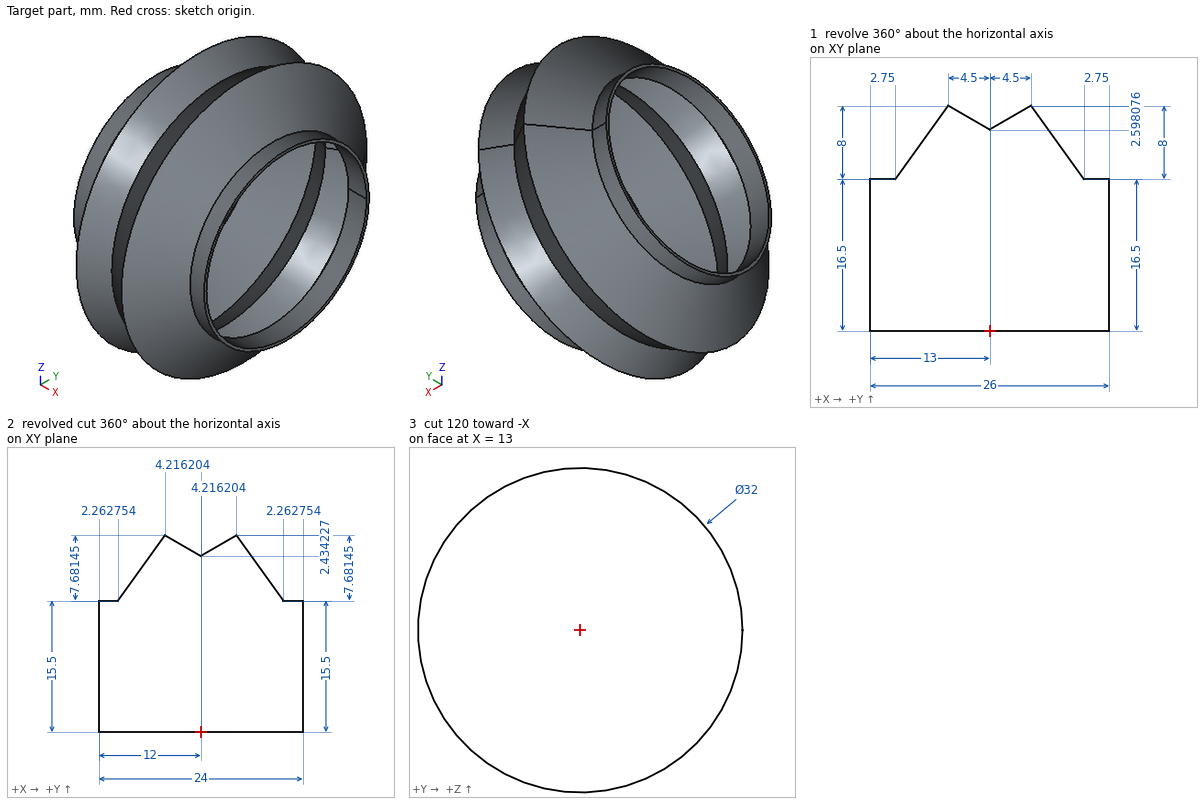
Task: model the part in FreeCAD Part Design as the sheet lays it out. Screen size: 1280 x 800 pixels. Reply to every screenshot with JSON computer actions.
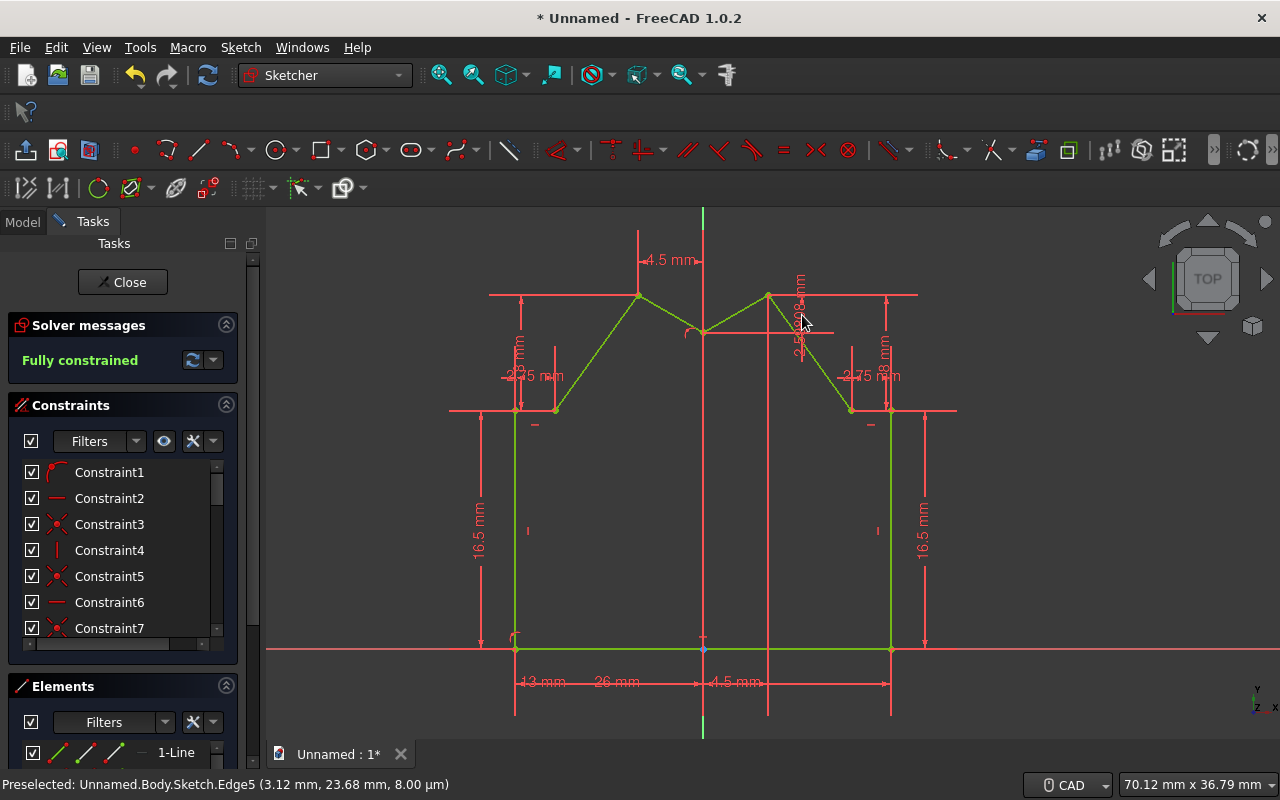
{"action": "left_click", "coordinate": [123, 282]}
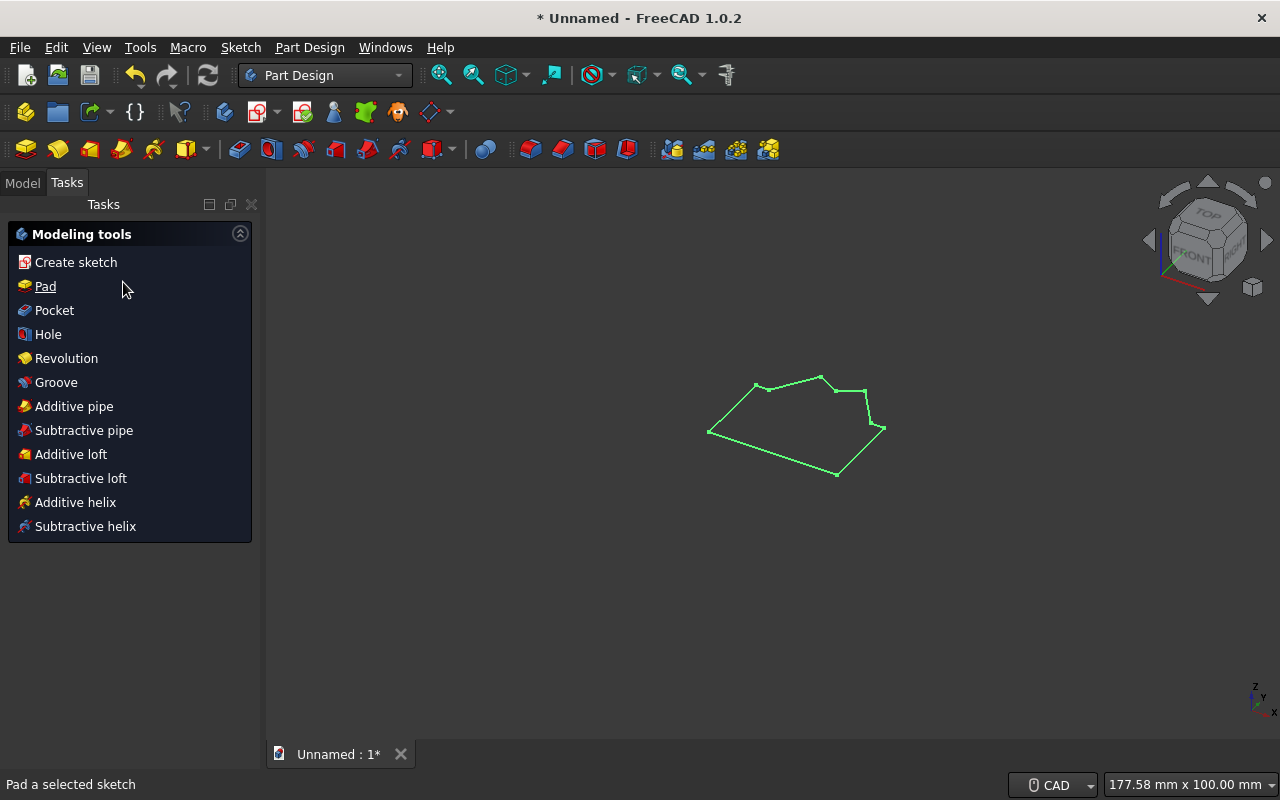
{"action": "left_click", "coordinate": [58, 150]}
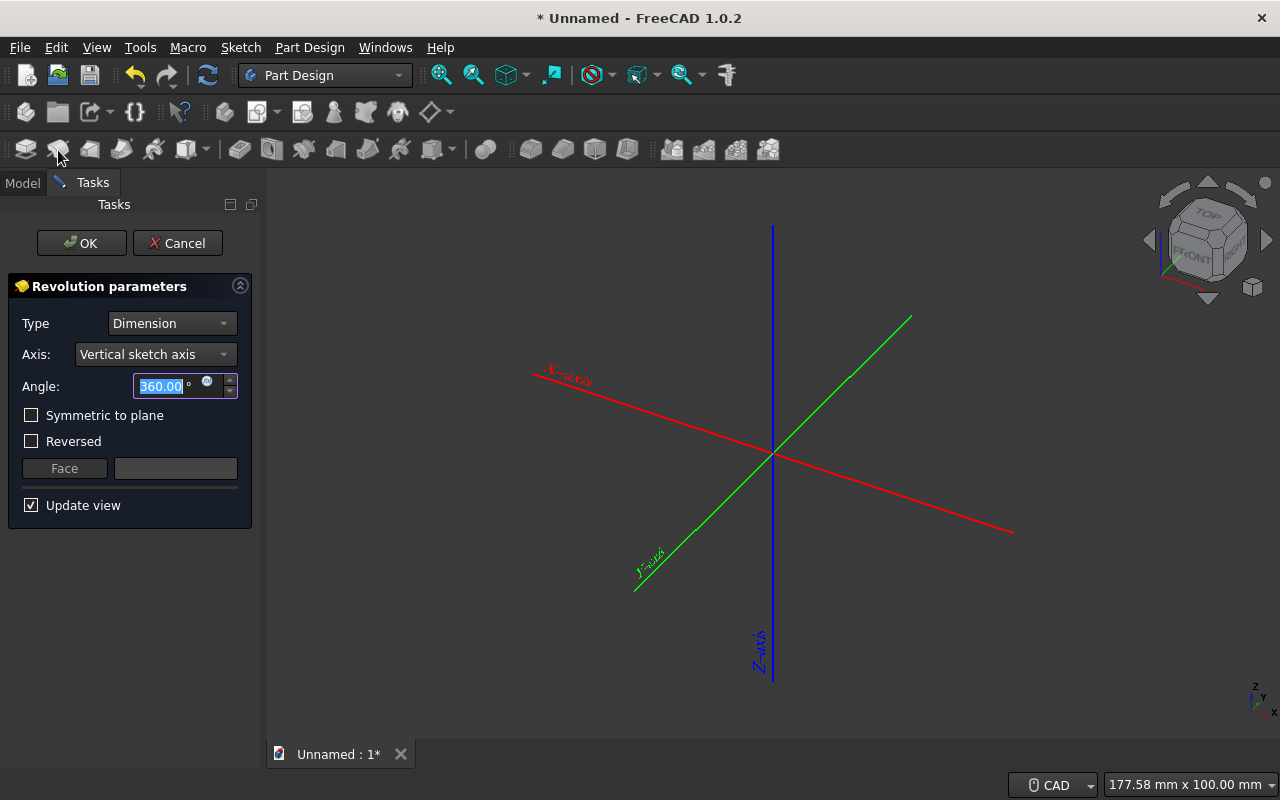
{"action": "left_click", "coordinate": [156, 354]}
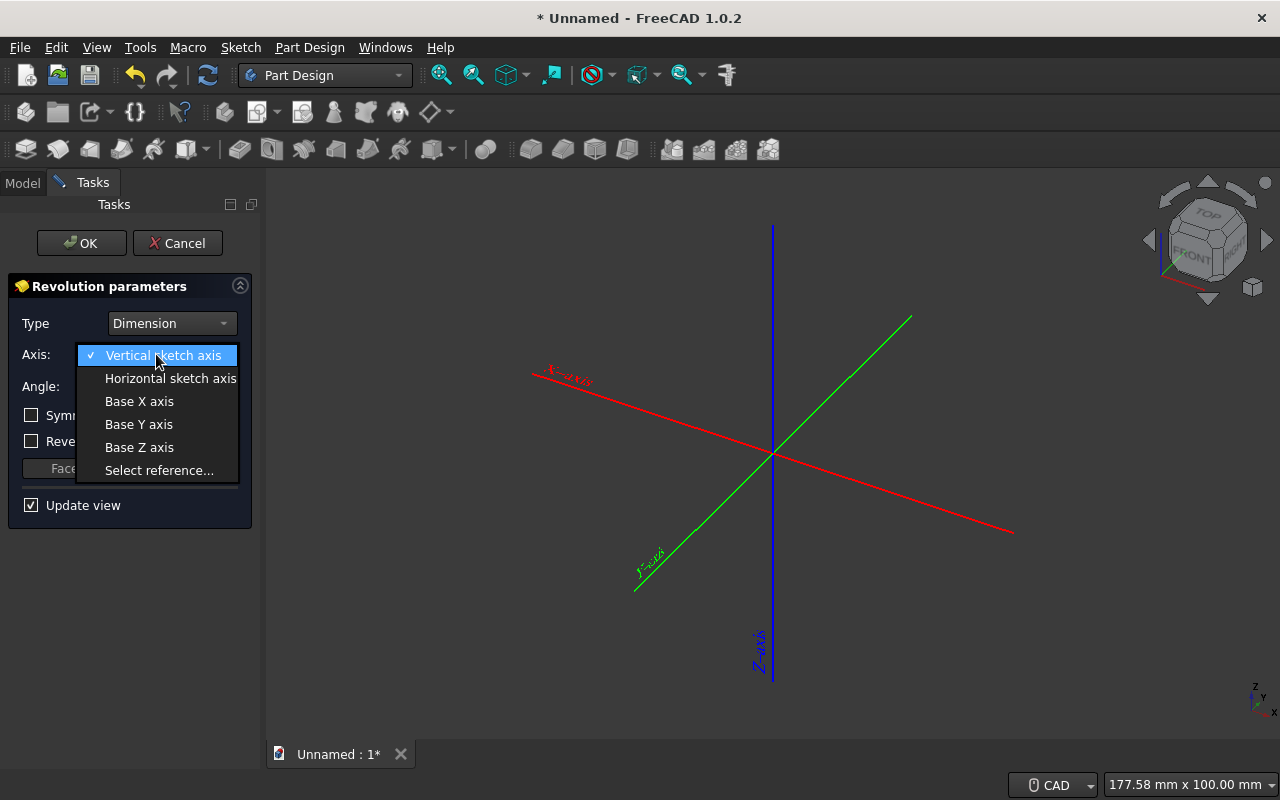
{"action": "left_click", "coordinate": [156, 378]}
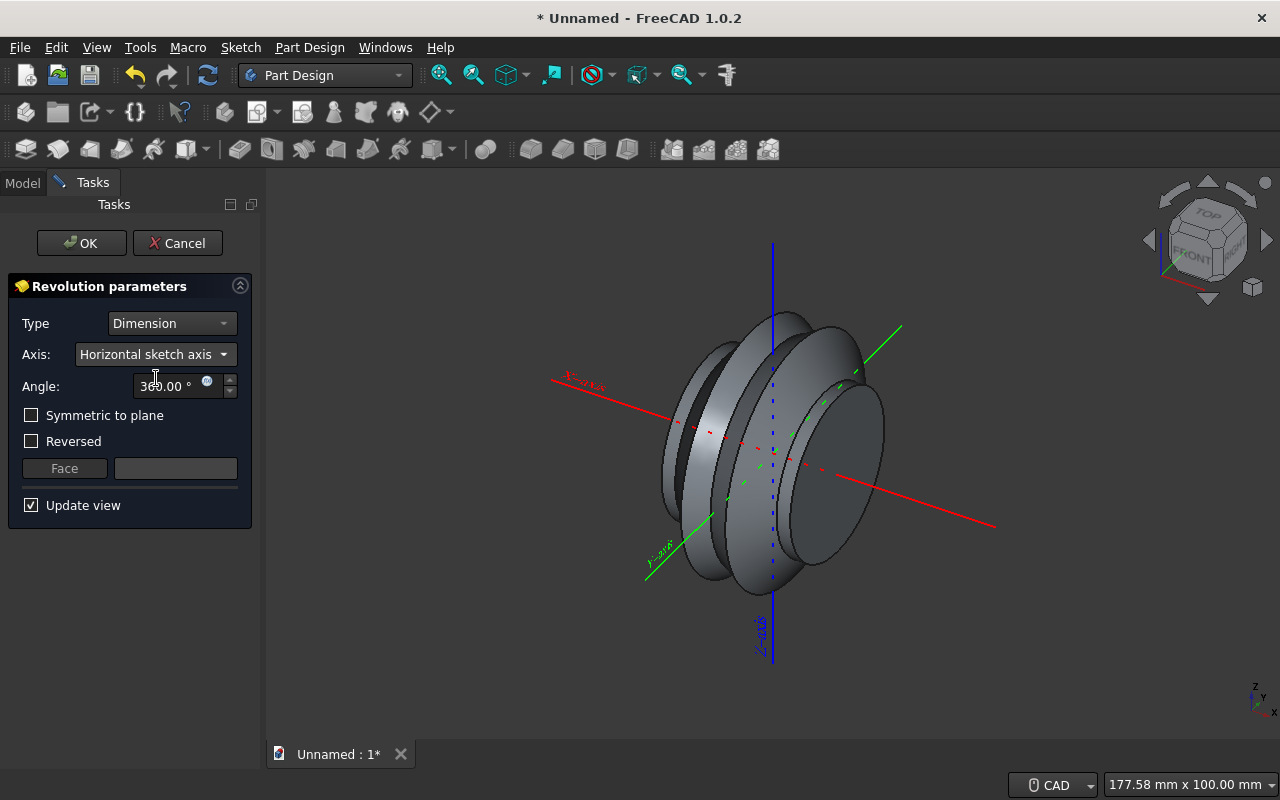
{"action": "left_click", "coordinate": [82, 243]}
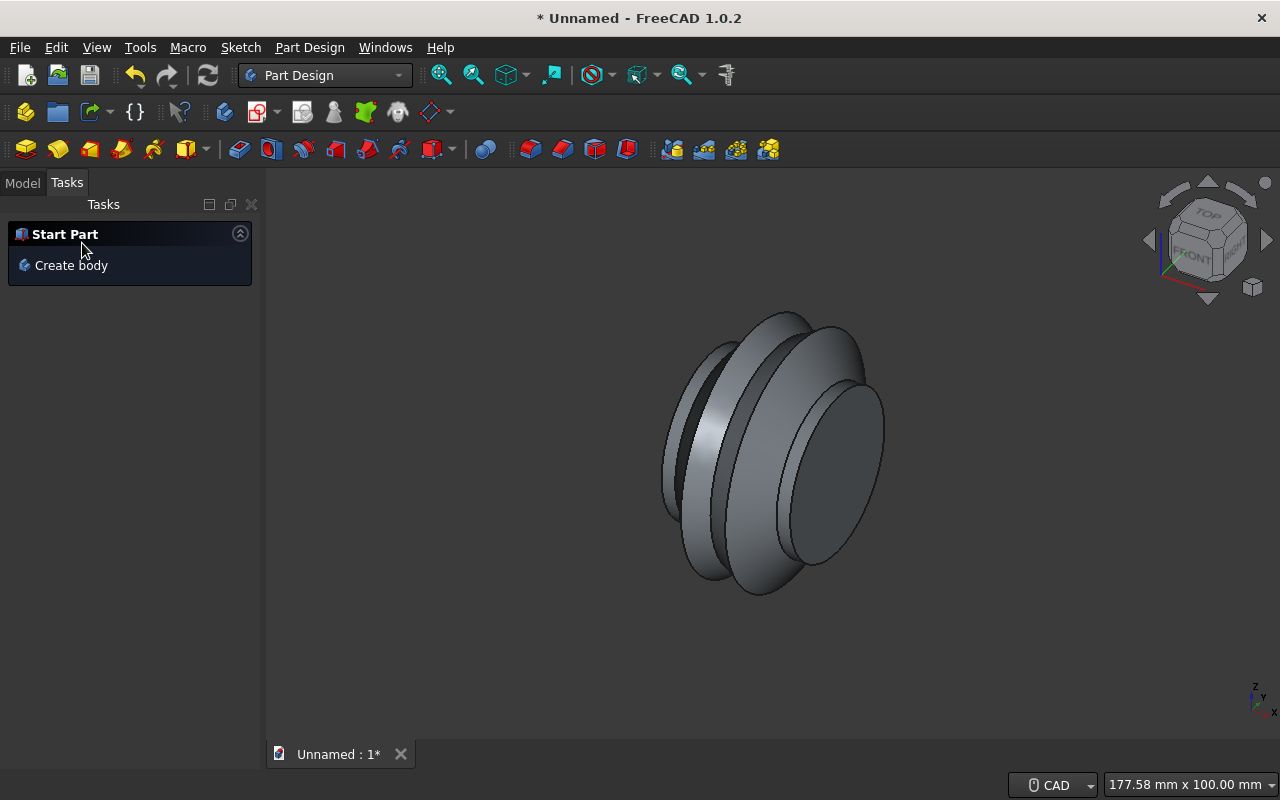
{"action": "left_click", "coordinate": [258, 112]}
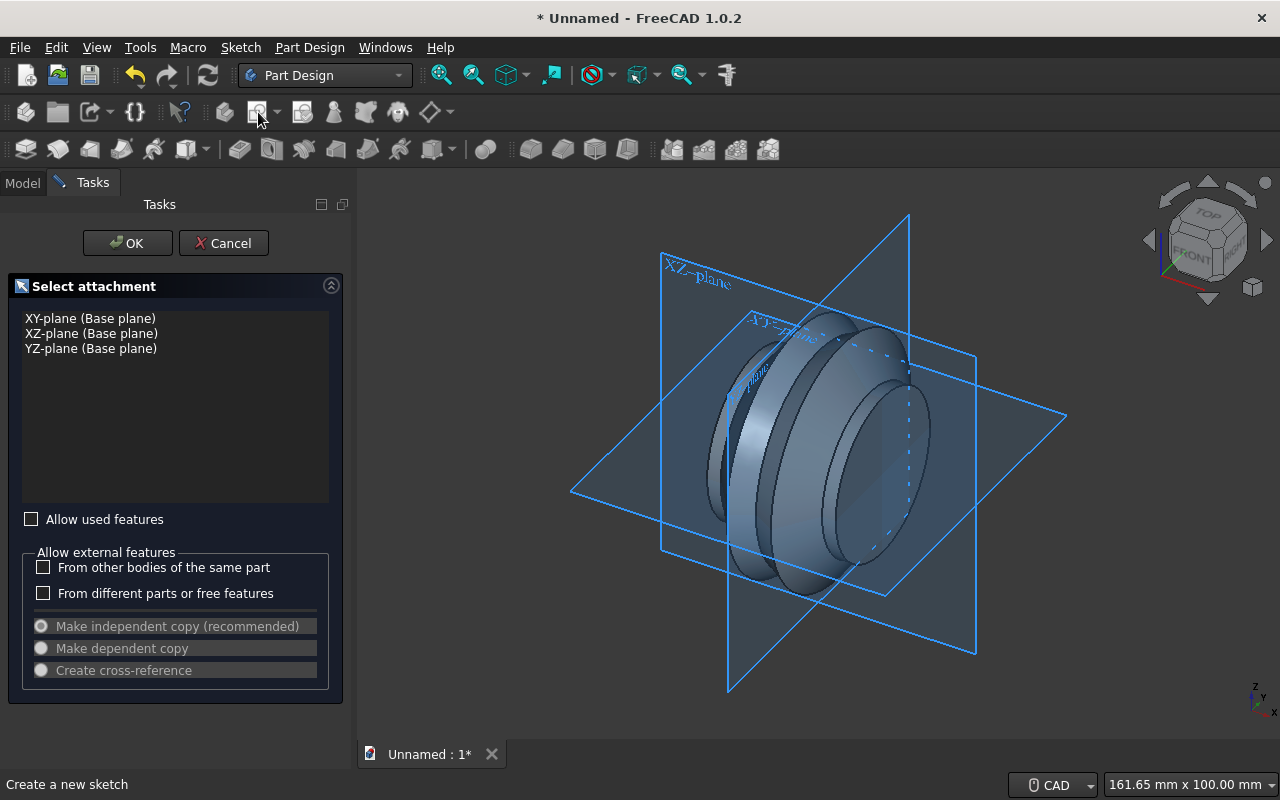
{"action": "left_click", "coordinate": [82, 318]}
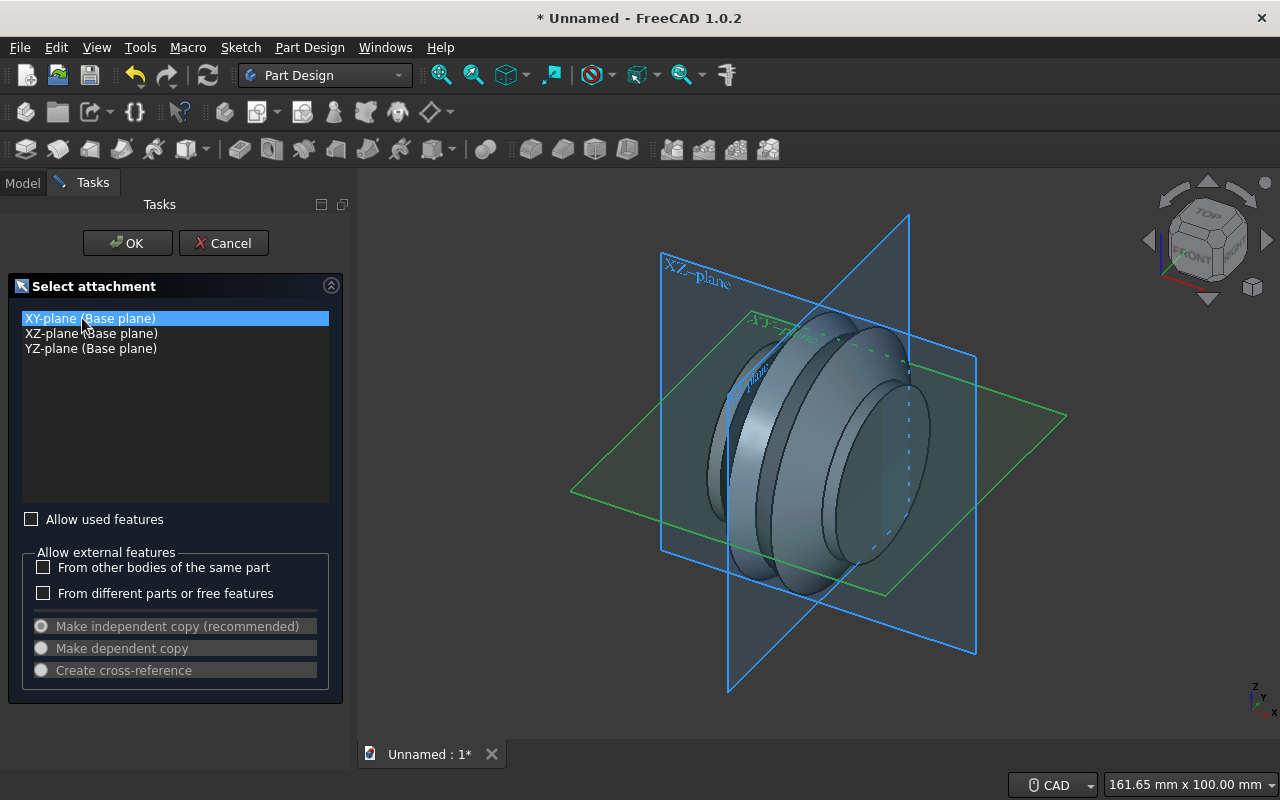
{"action": "left_click", "coordinate": [128, 243]}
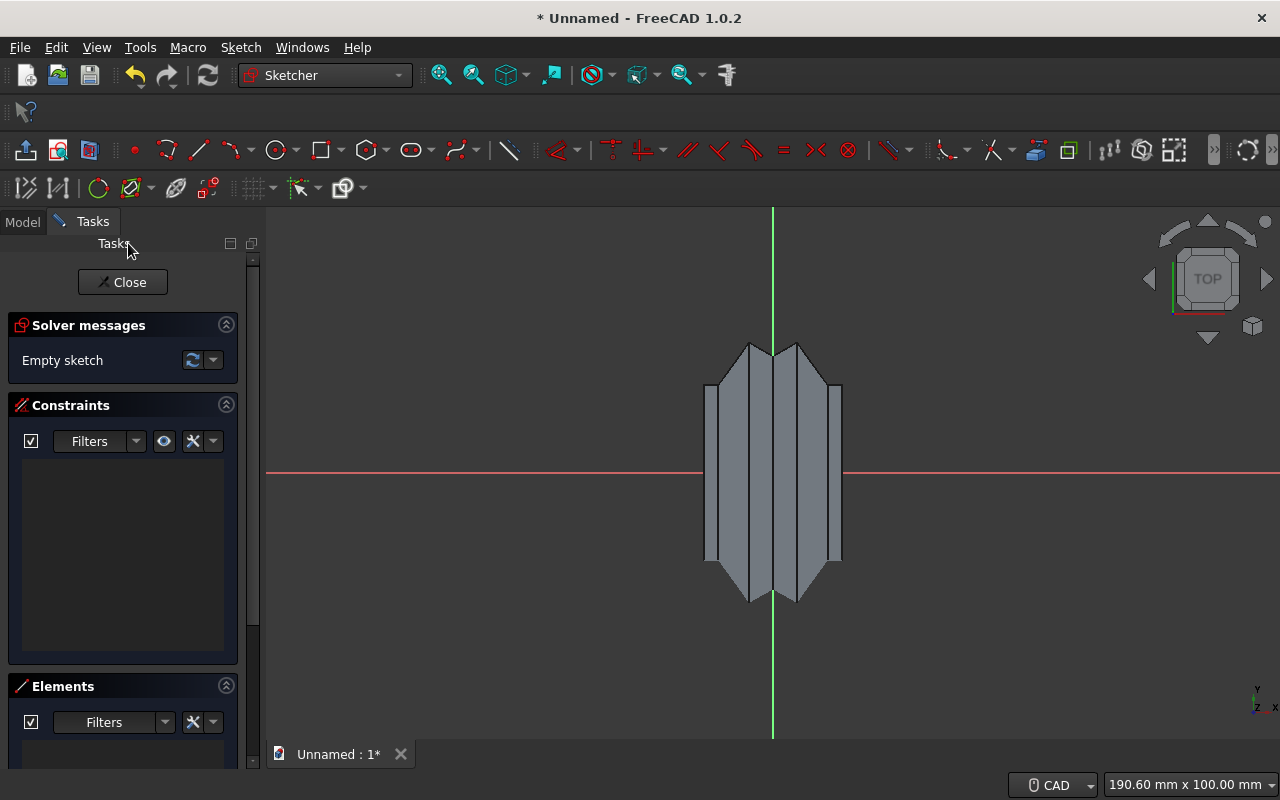
{"action": "key", "text": "q s"}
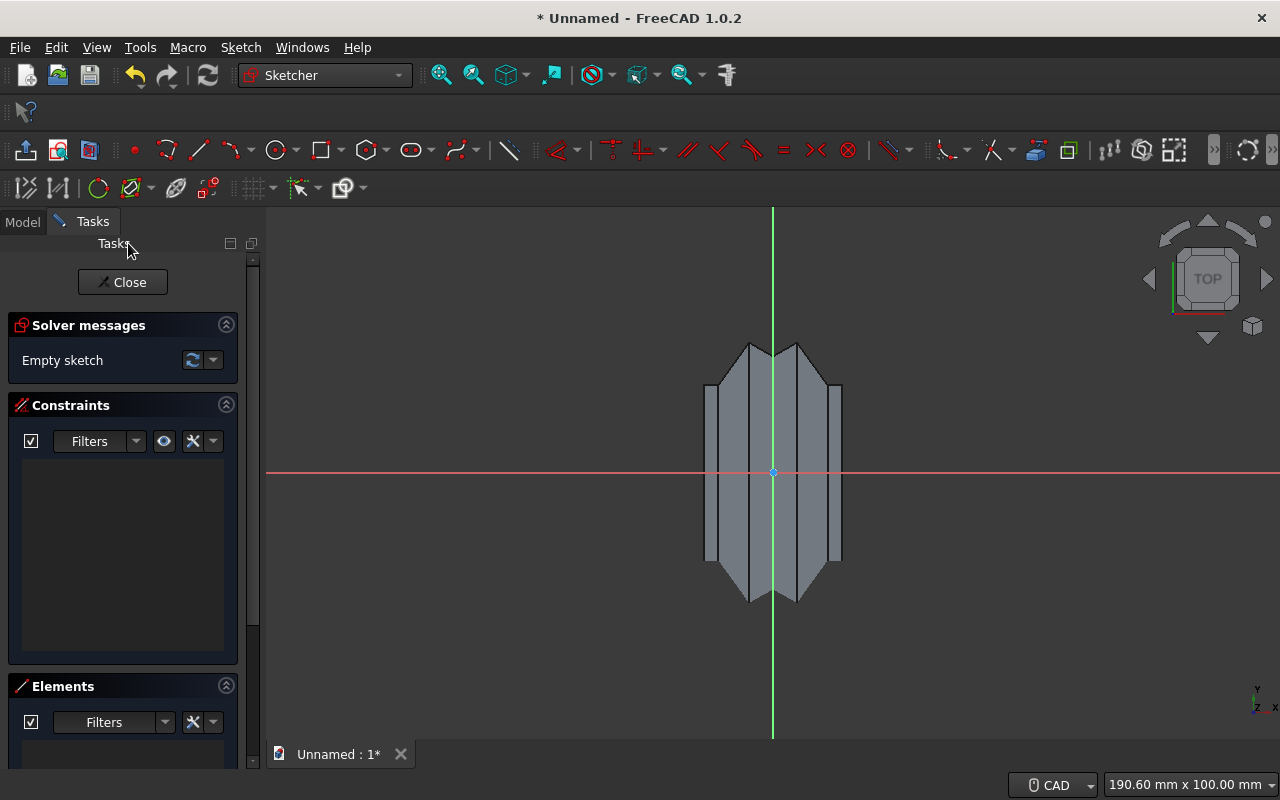
{"action": "scroll", "coordinate": [813, 375], "scroll_direction": "up", "scroll_amount": 5}